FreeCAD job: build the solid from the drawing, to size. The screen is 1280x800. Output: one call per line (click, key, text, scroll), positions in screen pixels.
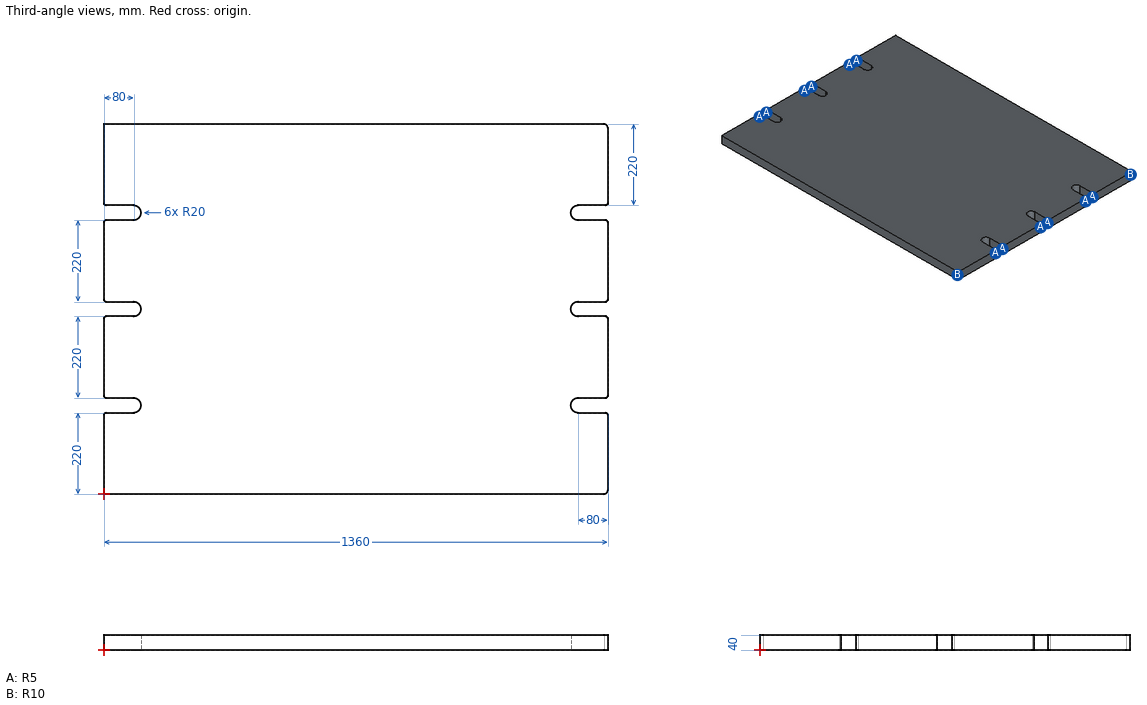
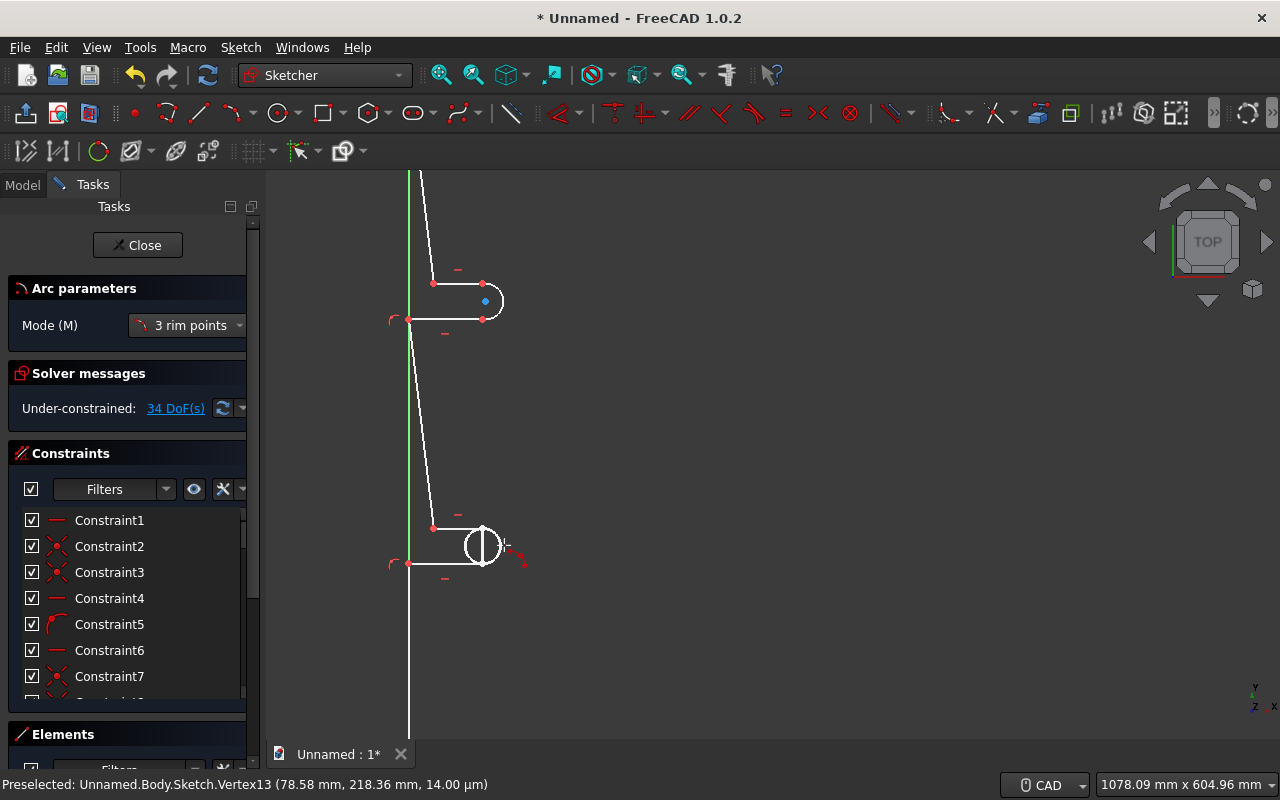
click(503, 544)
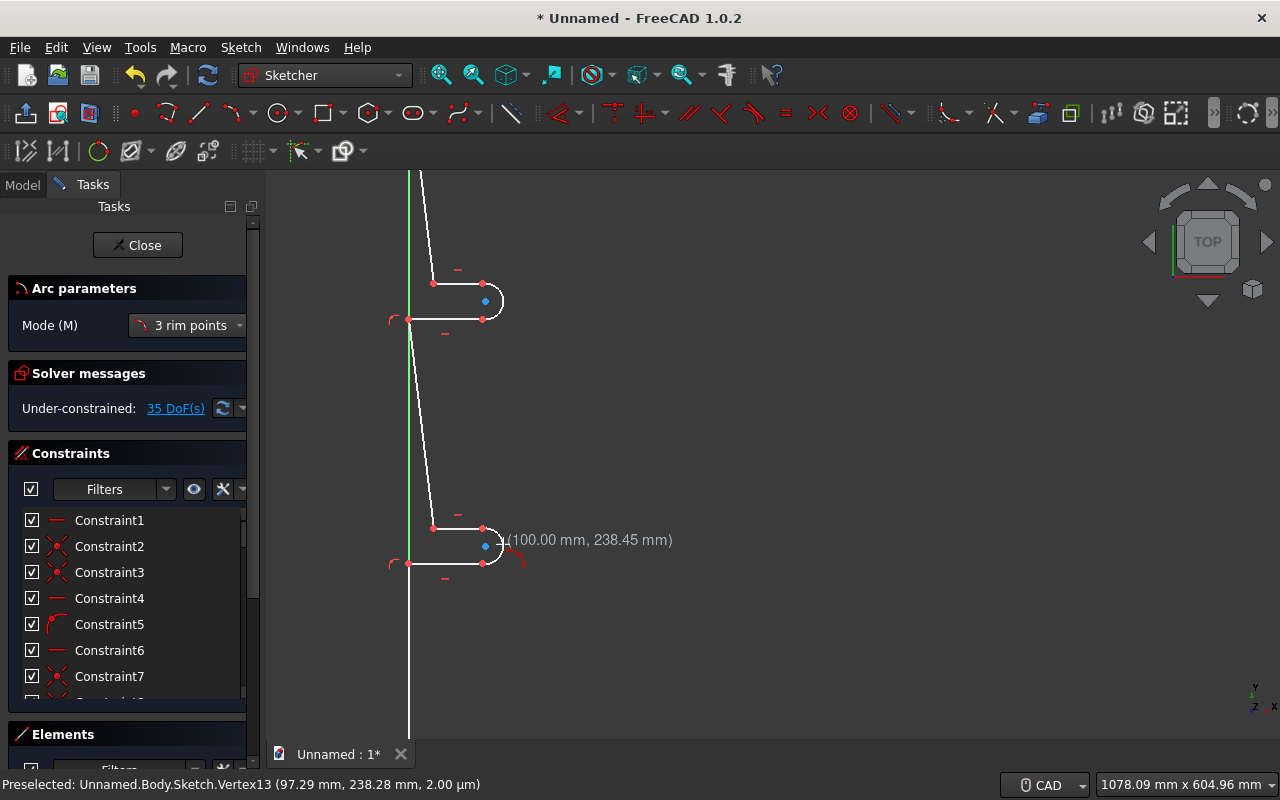
scroll(504, 545, down, 5)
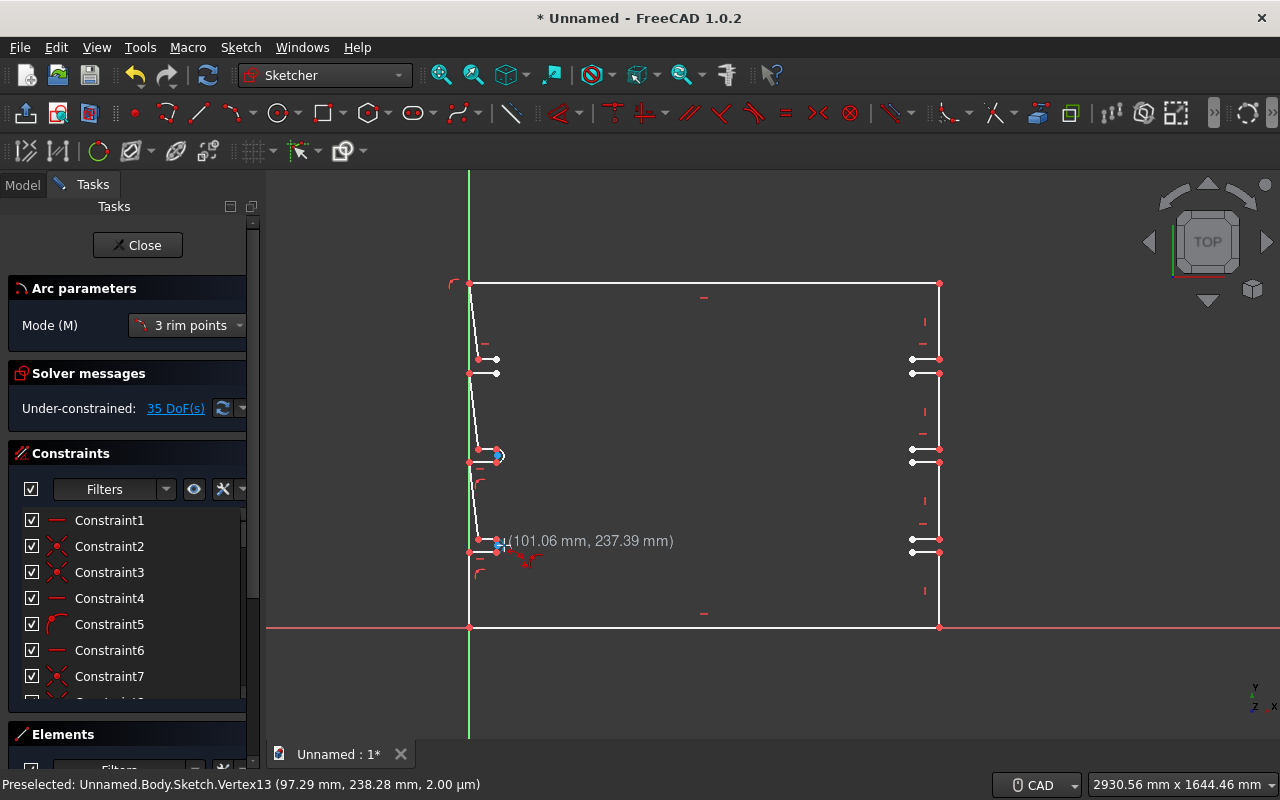
click(912, 552)
click(912, 539)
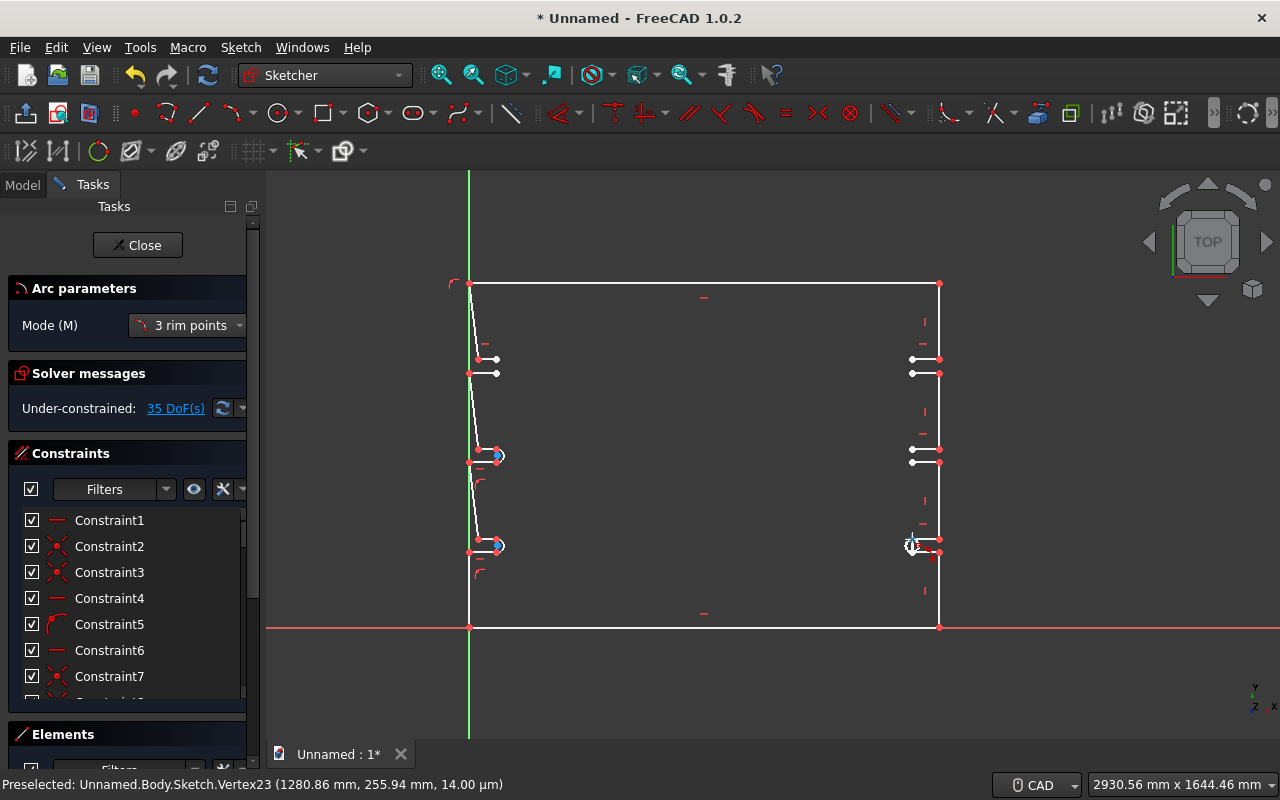
scroll(905, 545, up, 5)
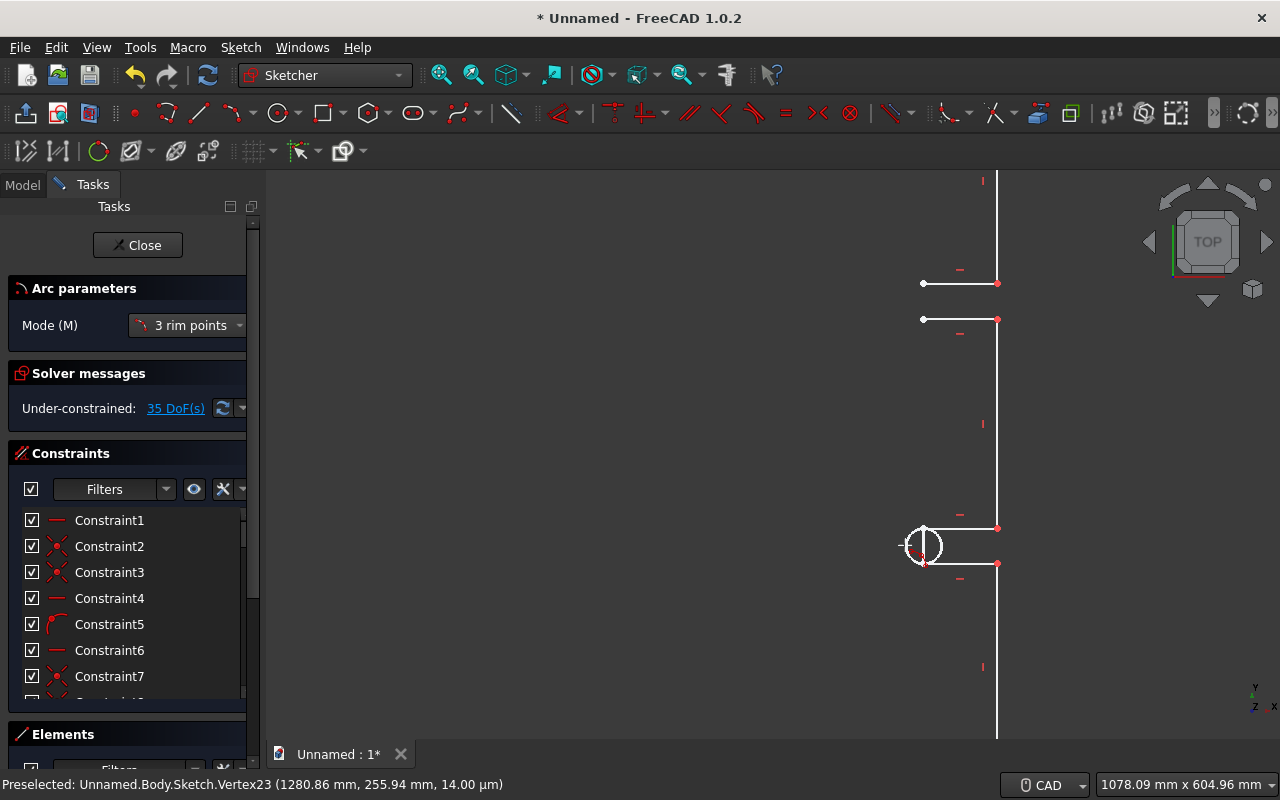
click(904, 544)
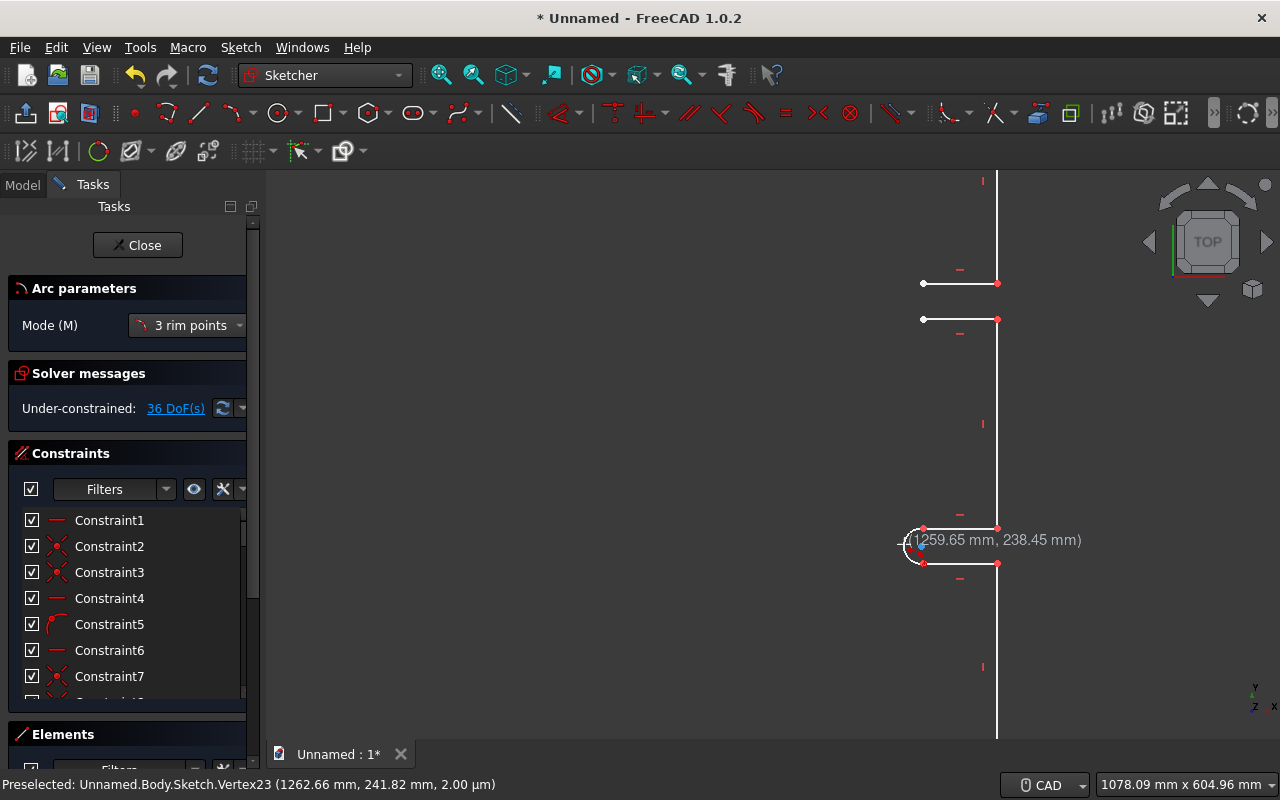
click(924, 319)
click(924, 284)
click(904, 299)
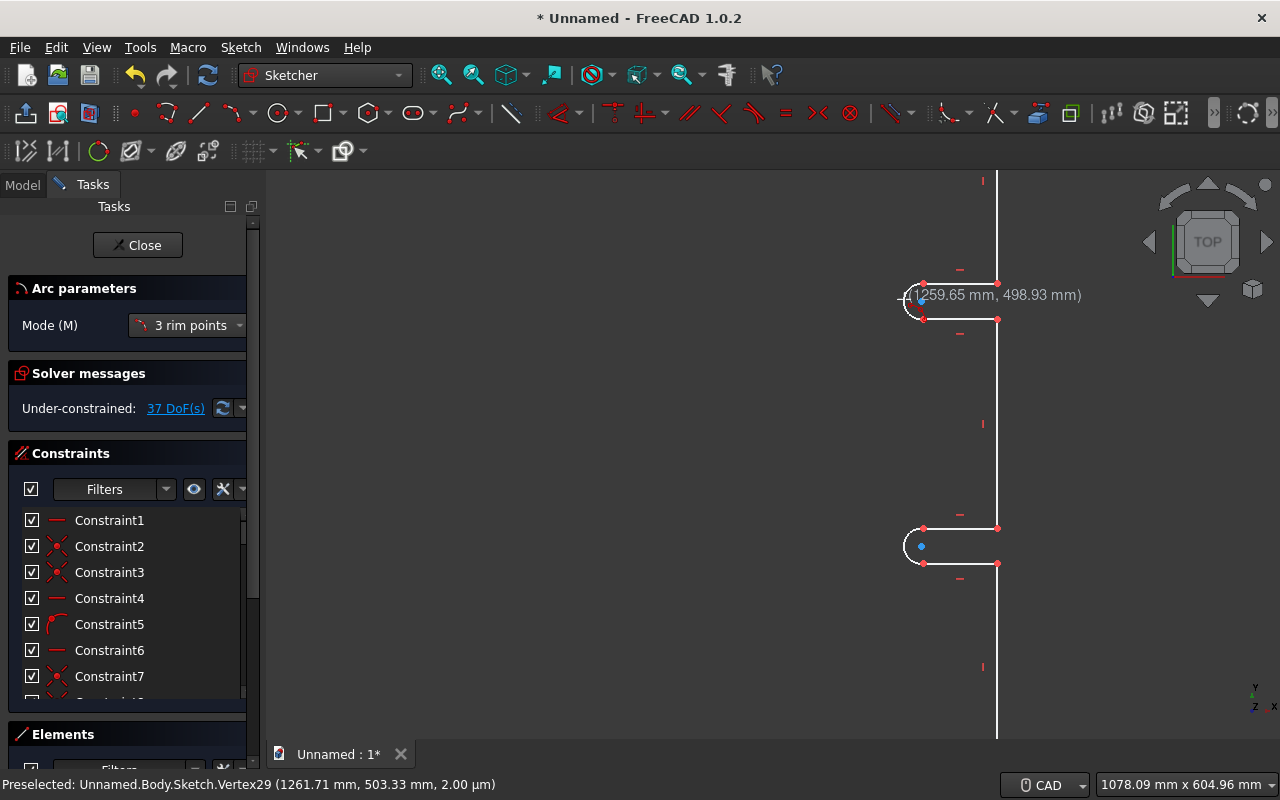
scroll(906, 545, down, 5)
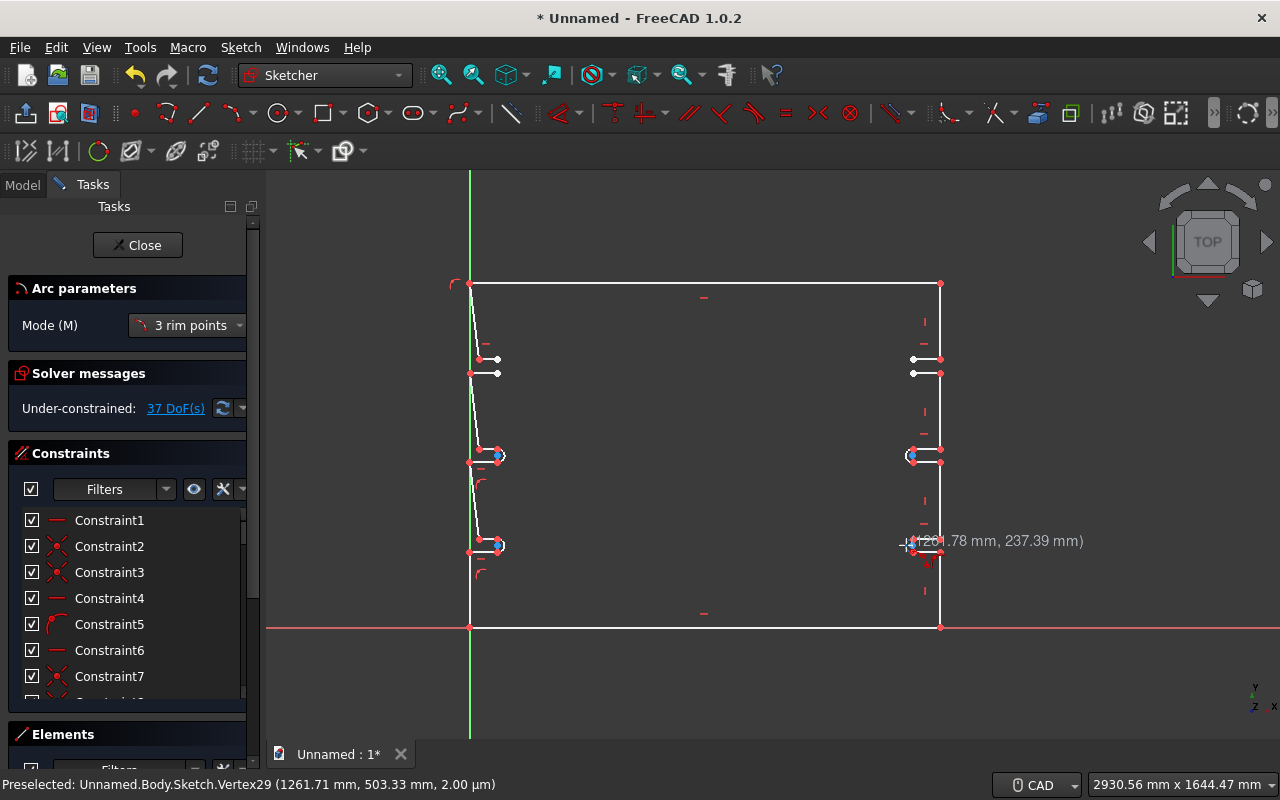
click(913, 373)
click(913, 359)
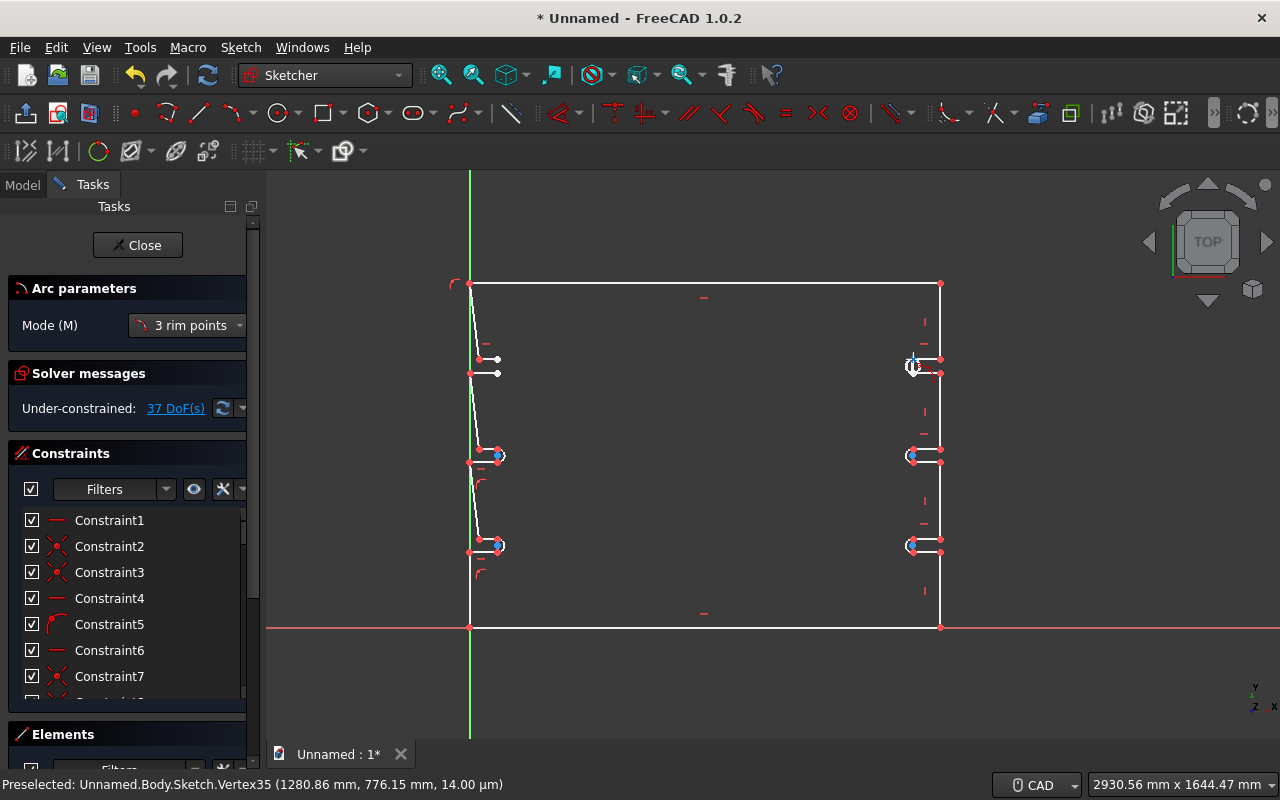
scroll(906, 365, up, 5)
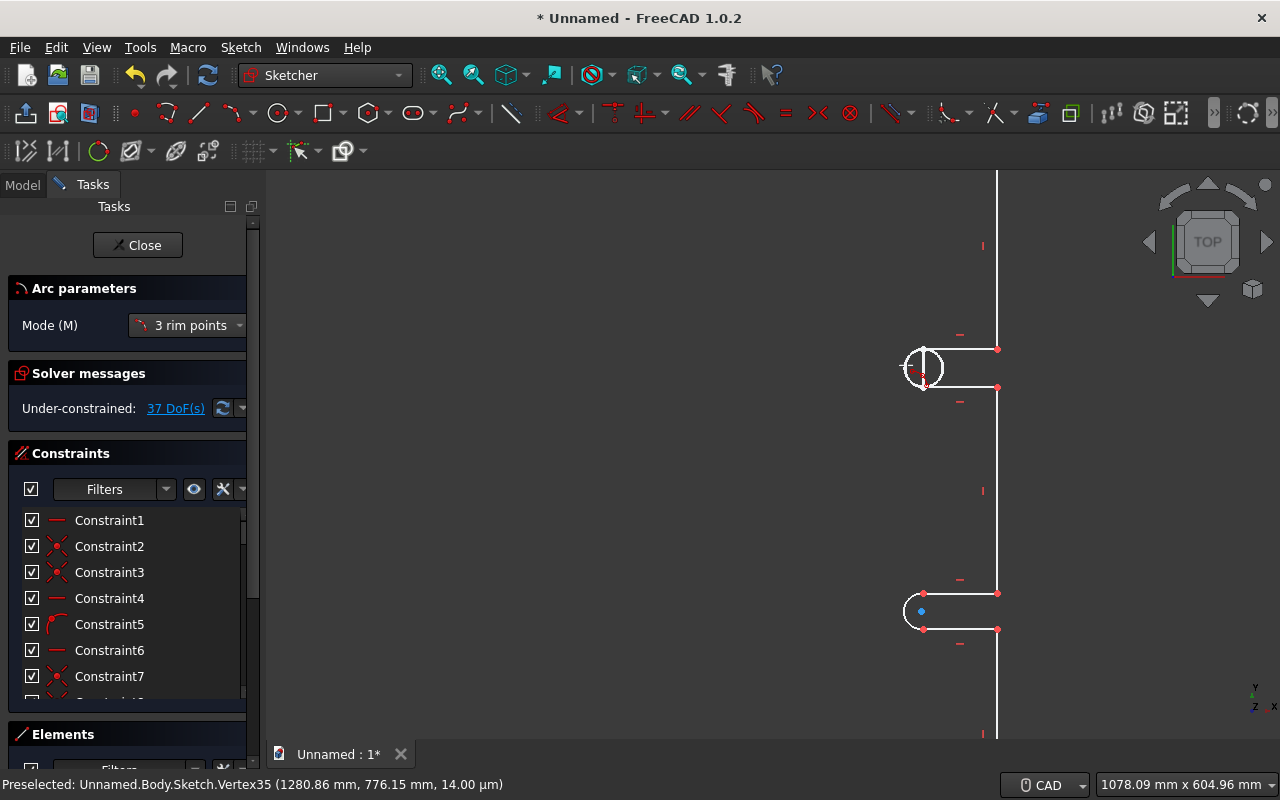
click(904, 364)